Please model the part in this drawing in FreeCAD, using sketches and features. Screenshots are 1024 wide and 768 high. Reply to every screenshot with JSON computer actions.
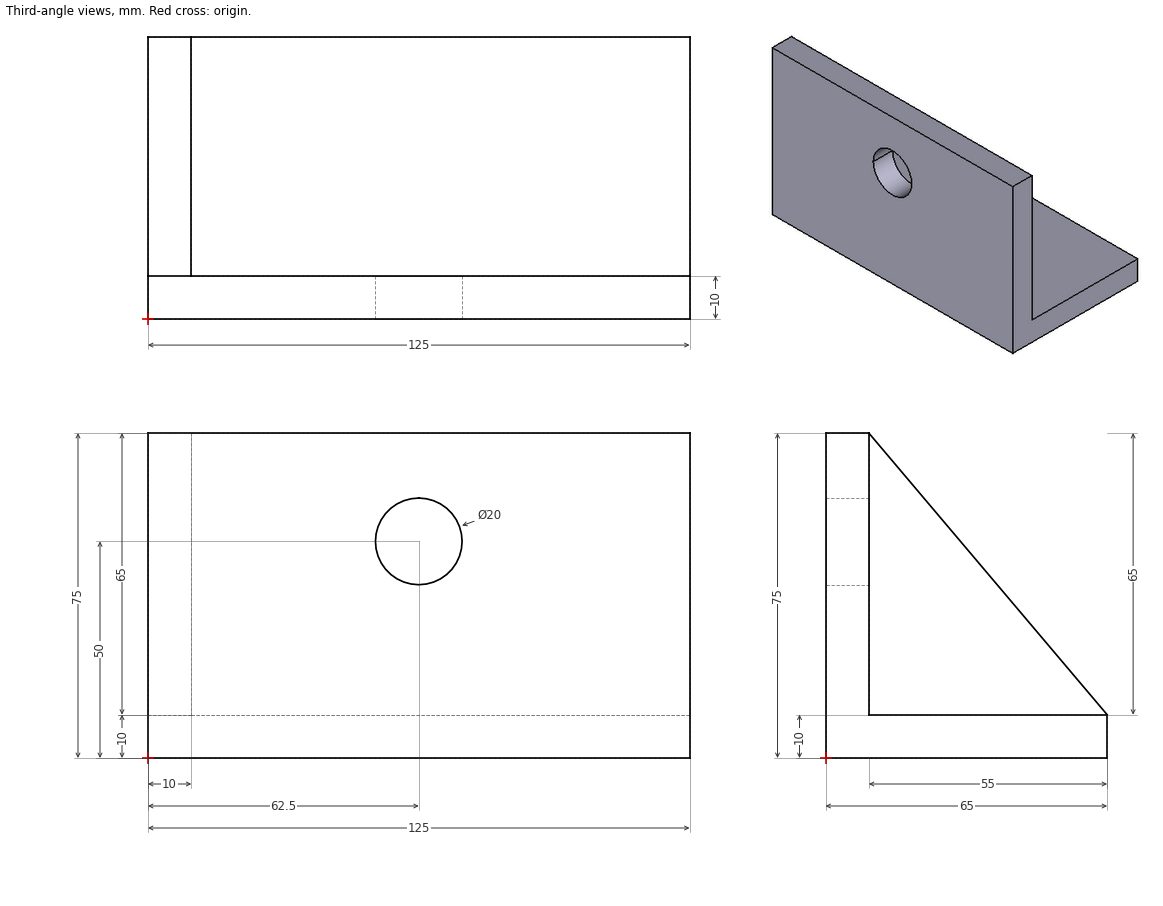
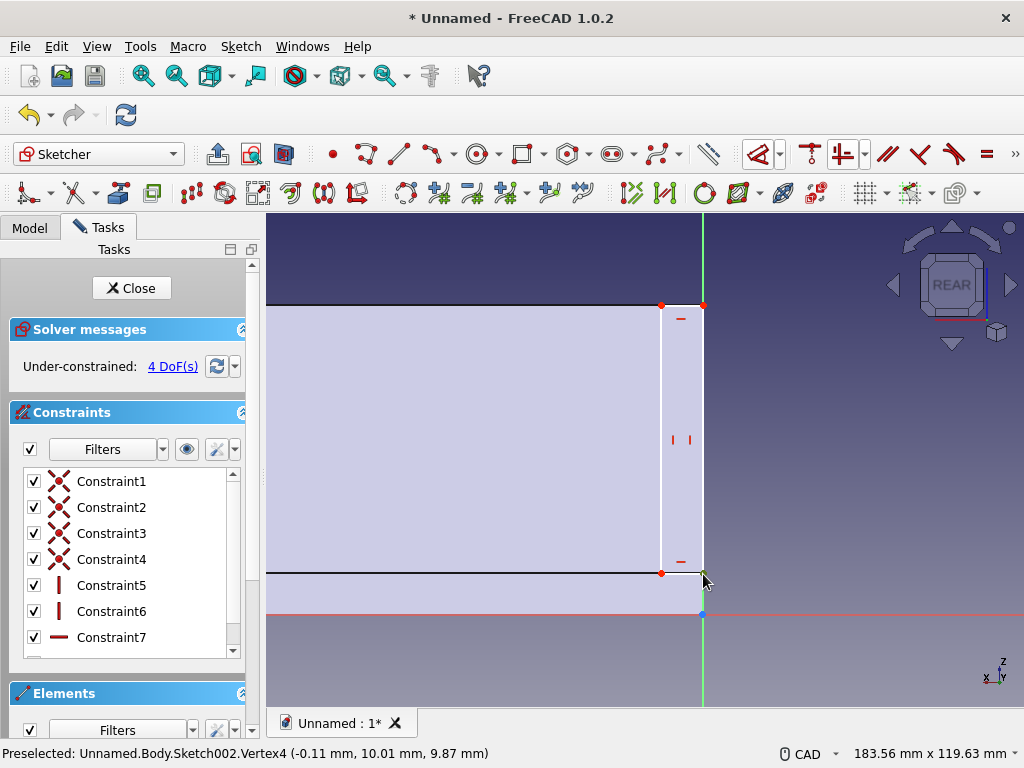
{"action": "left_click", "coordinate": [703, 648]}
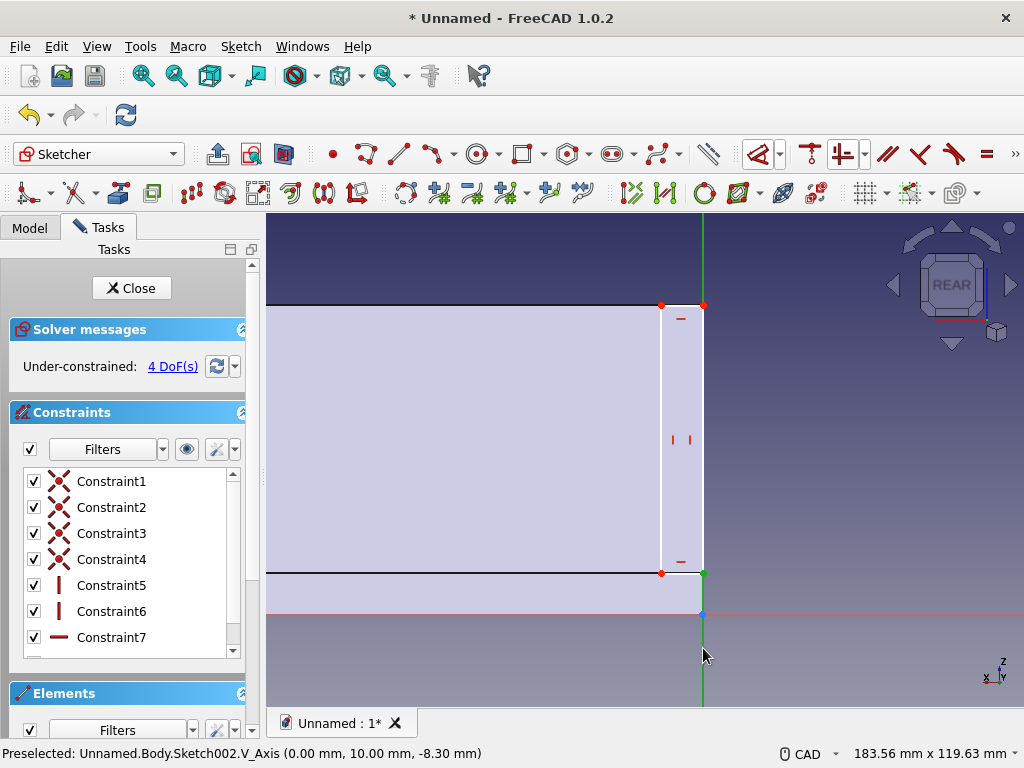
{"action": "left_click", "coordinate": [810, 154]}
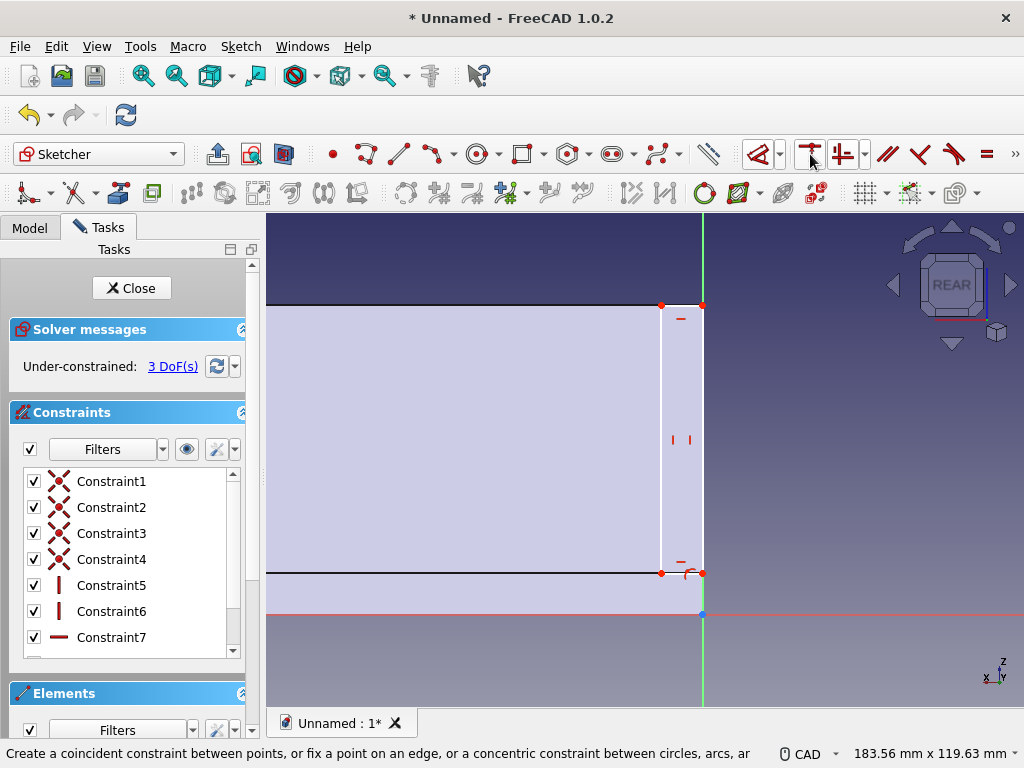
{"action": "left_click", "coordinate": [661, 386]}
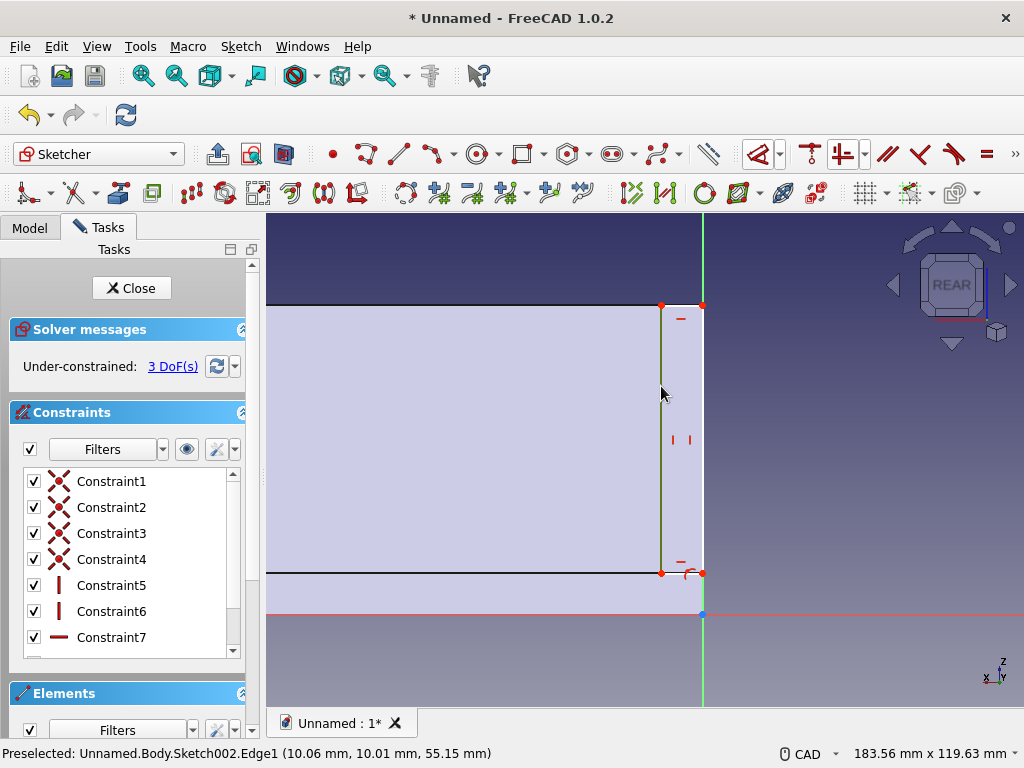
{"action": "key", "text": "i"}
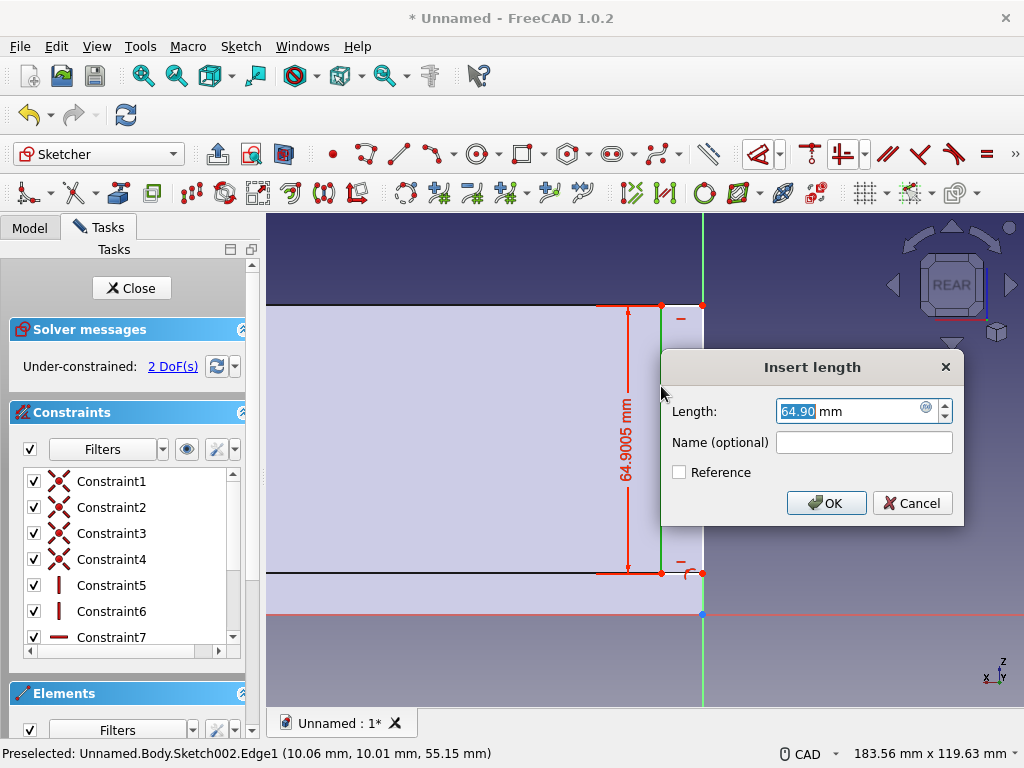
{"action": "type", "text": "65"}
{"action": "key", "text": "Return"}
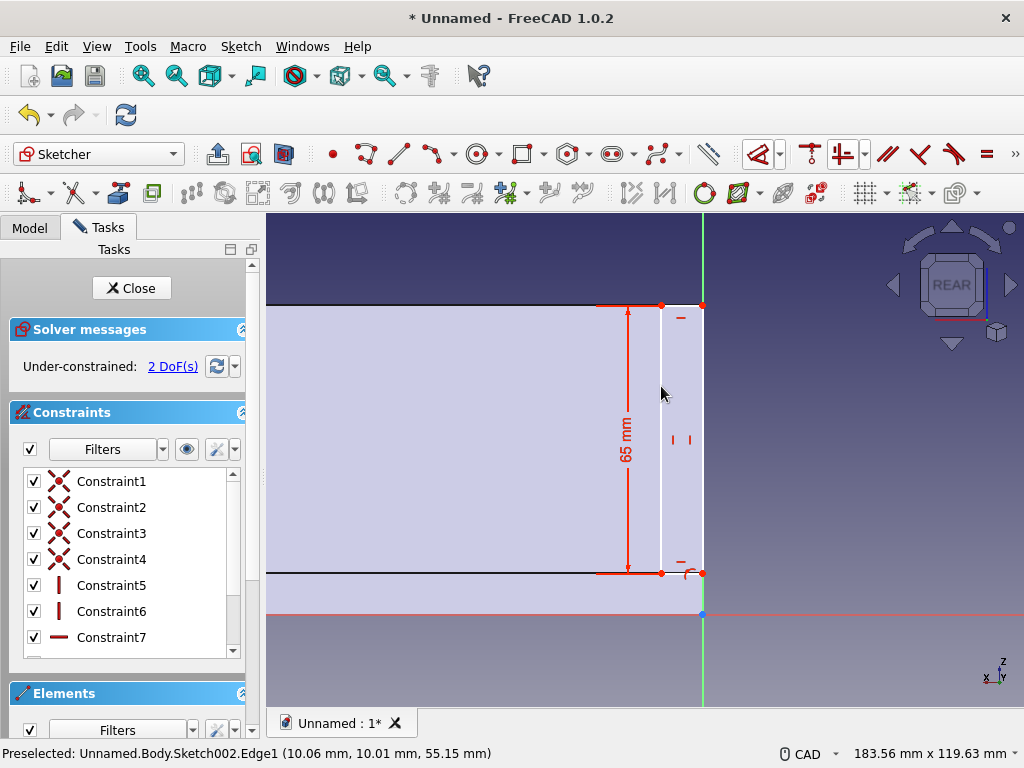
{"action": "left_click", "coordinate": [673, 574]}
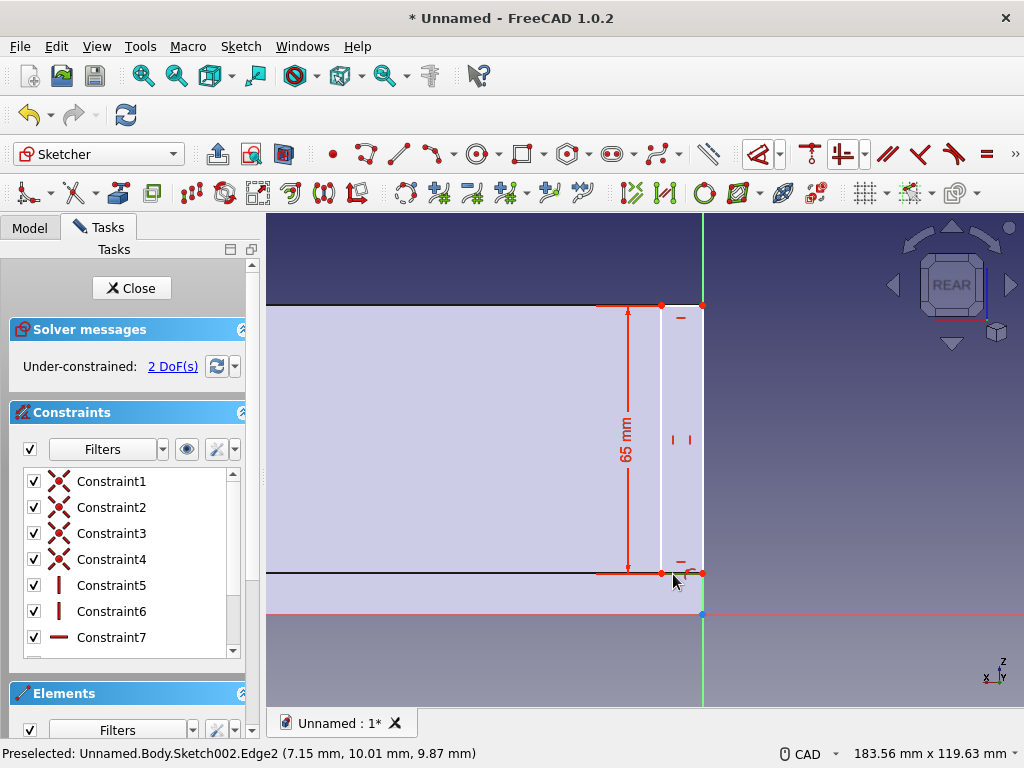
{"action": "key", "text": "l"}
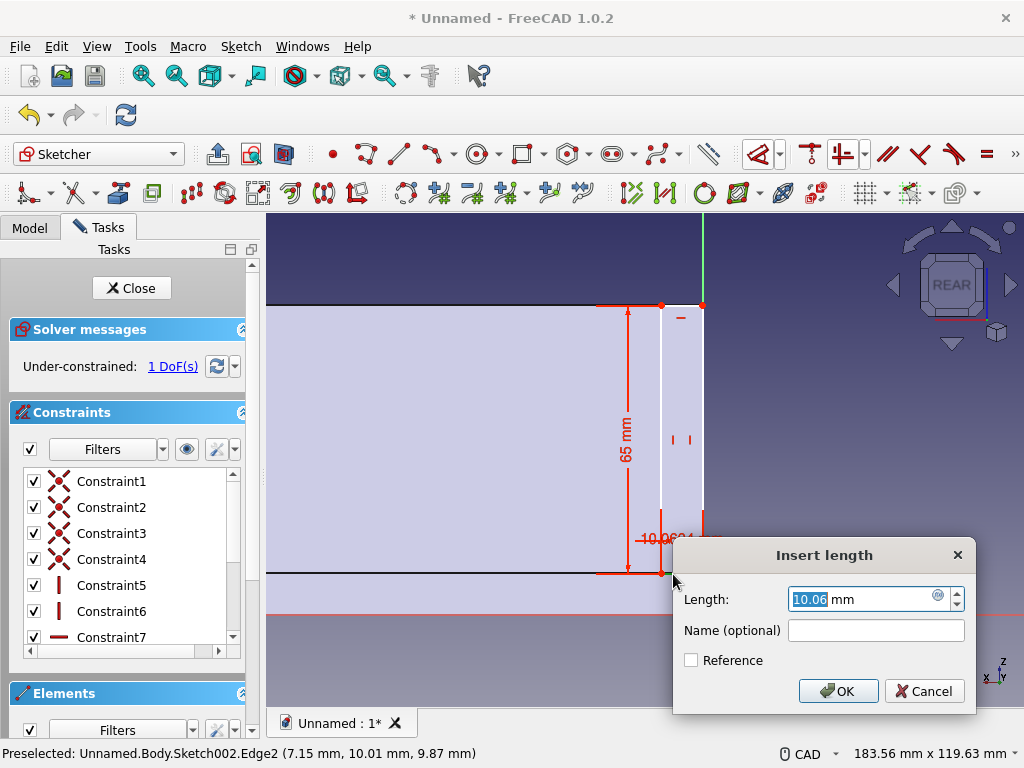
{"action": "type", "text": "10"}
{"action": "key", "text": "Return"}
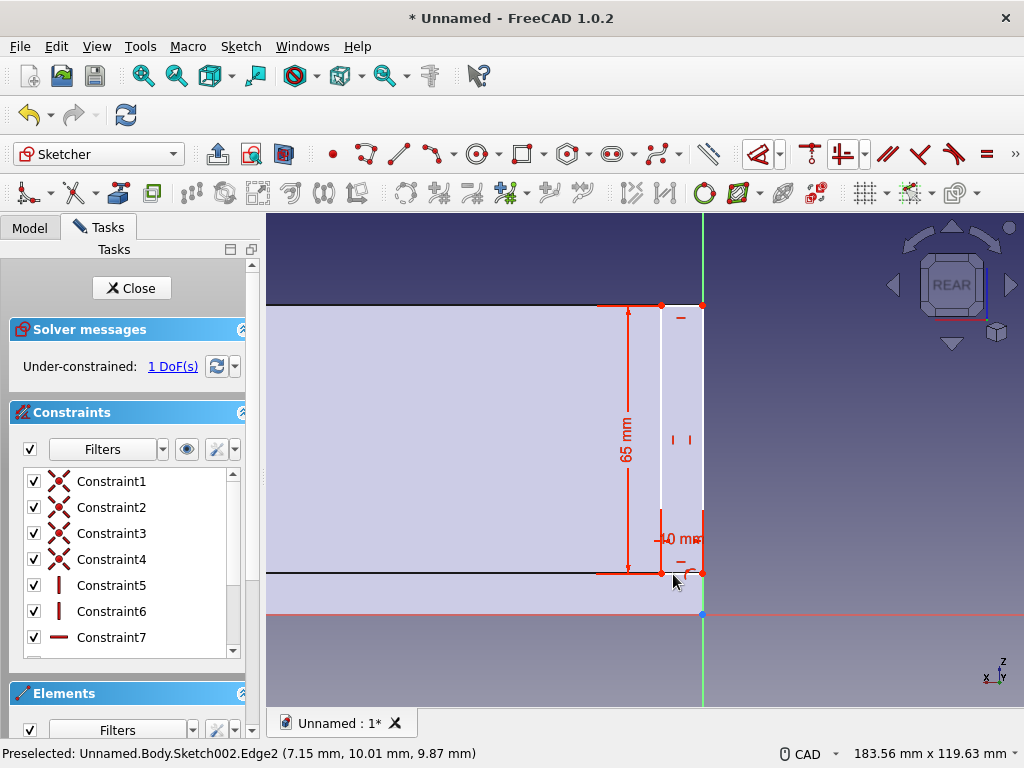
{"action": "left_click", "coordinate": [661, 306]}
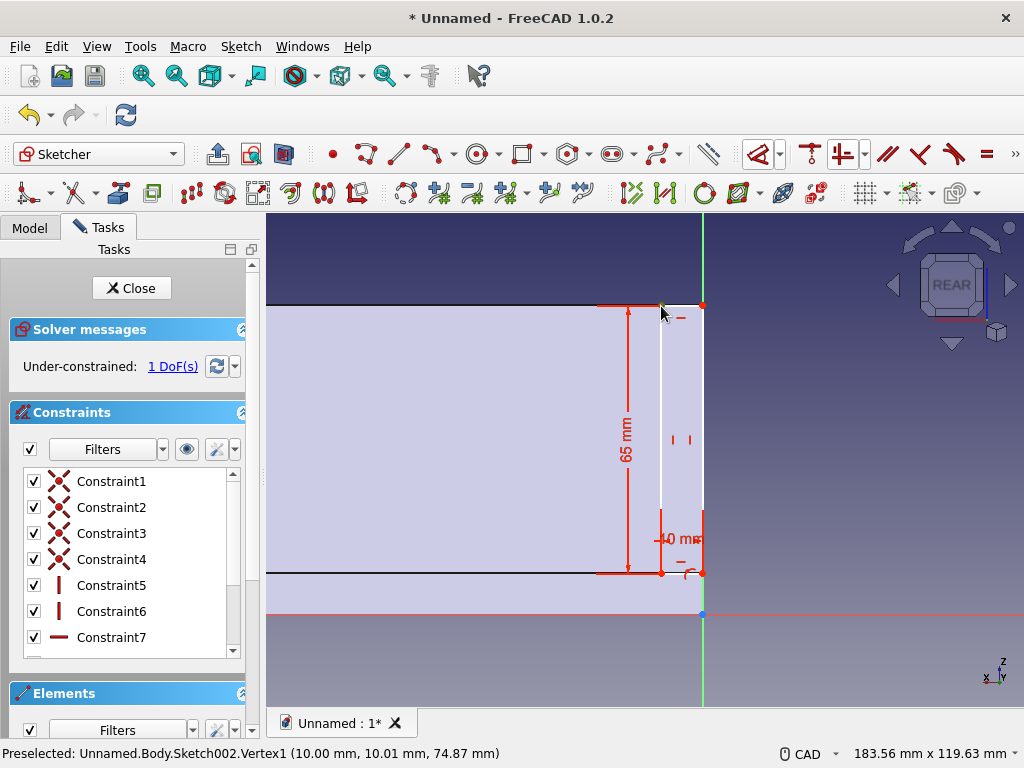
{"action": "left_click", "coordinate": [780, 154]}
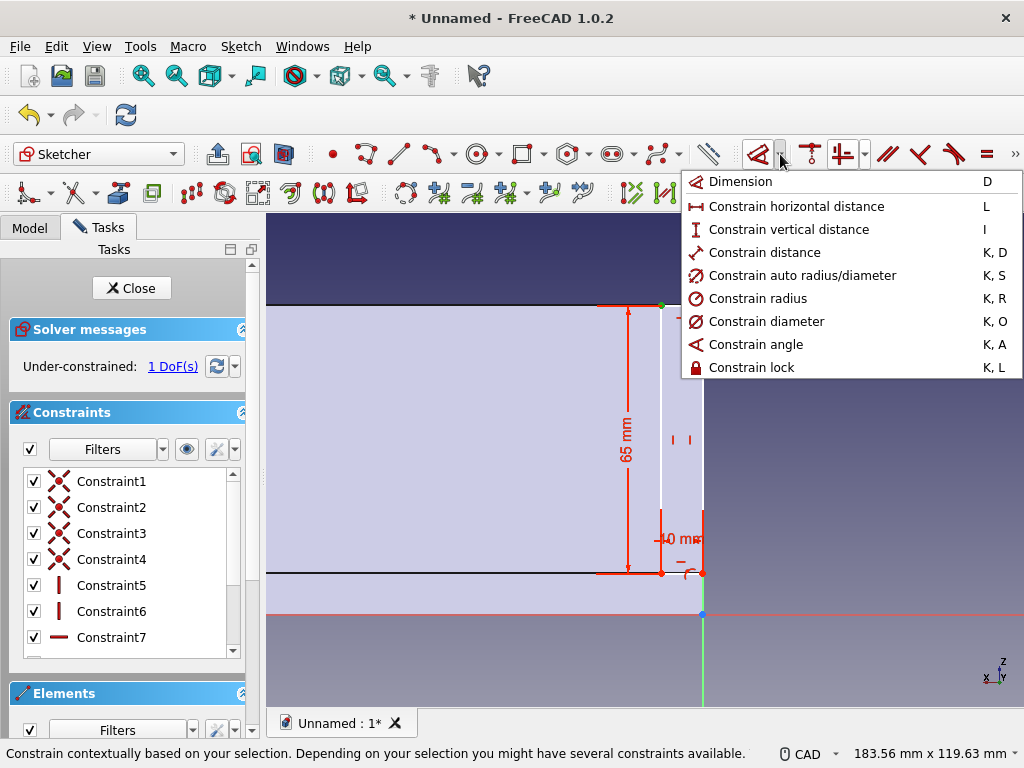
{"action": "left_click", "coordinate": [852, 230]}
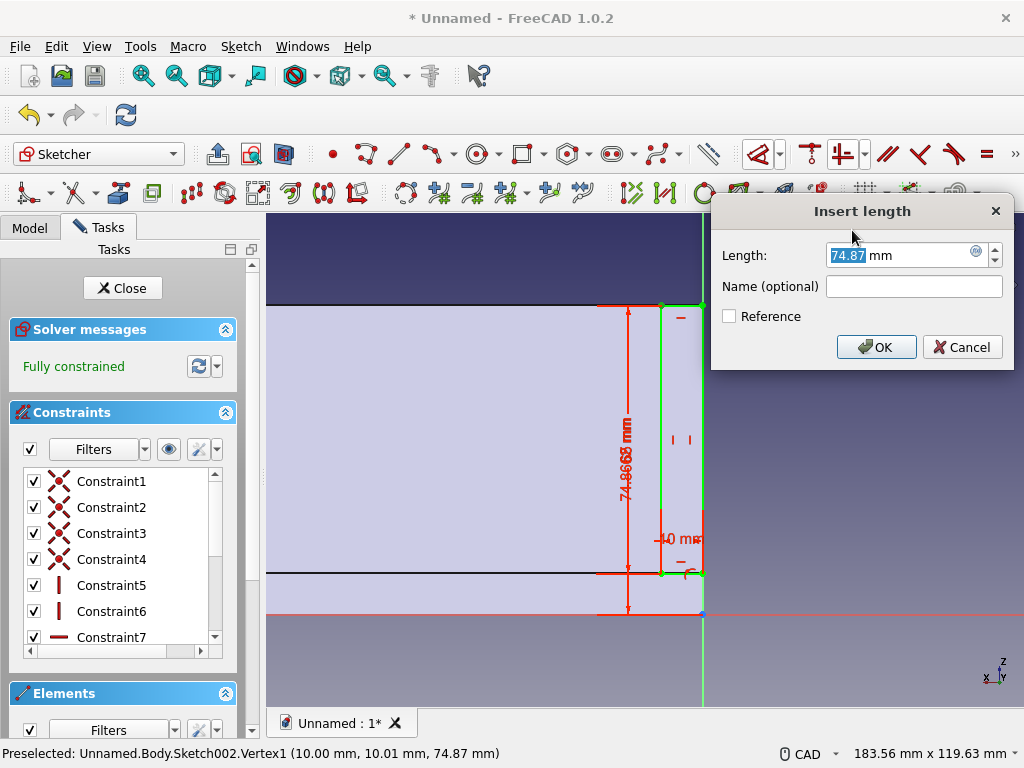
{"action": "type", "text": "75"}
{"action": "key", "text": "Return"}